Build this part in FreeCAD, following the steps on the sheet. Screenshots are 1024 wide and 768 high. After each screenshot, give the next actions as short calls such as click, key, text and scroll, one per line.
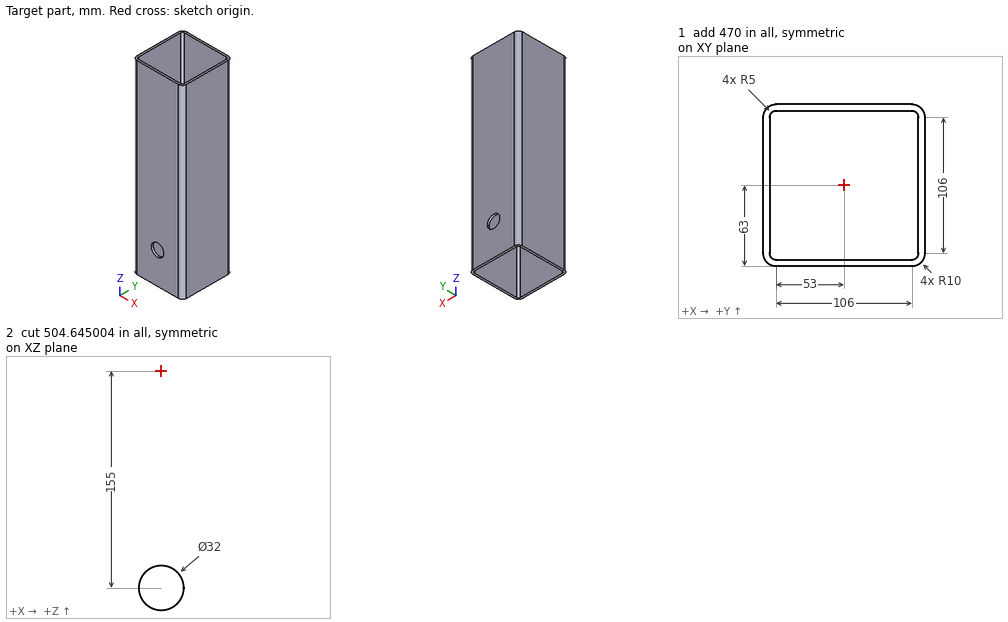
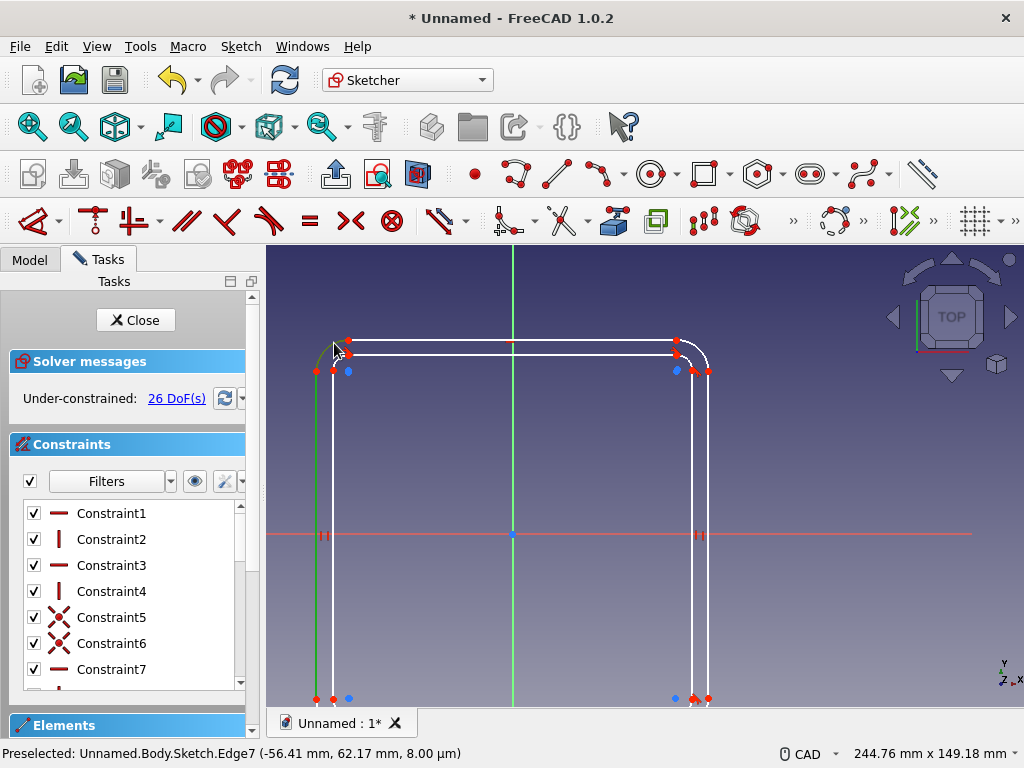
click(269, 222)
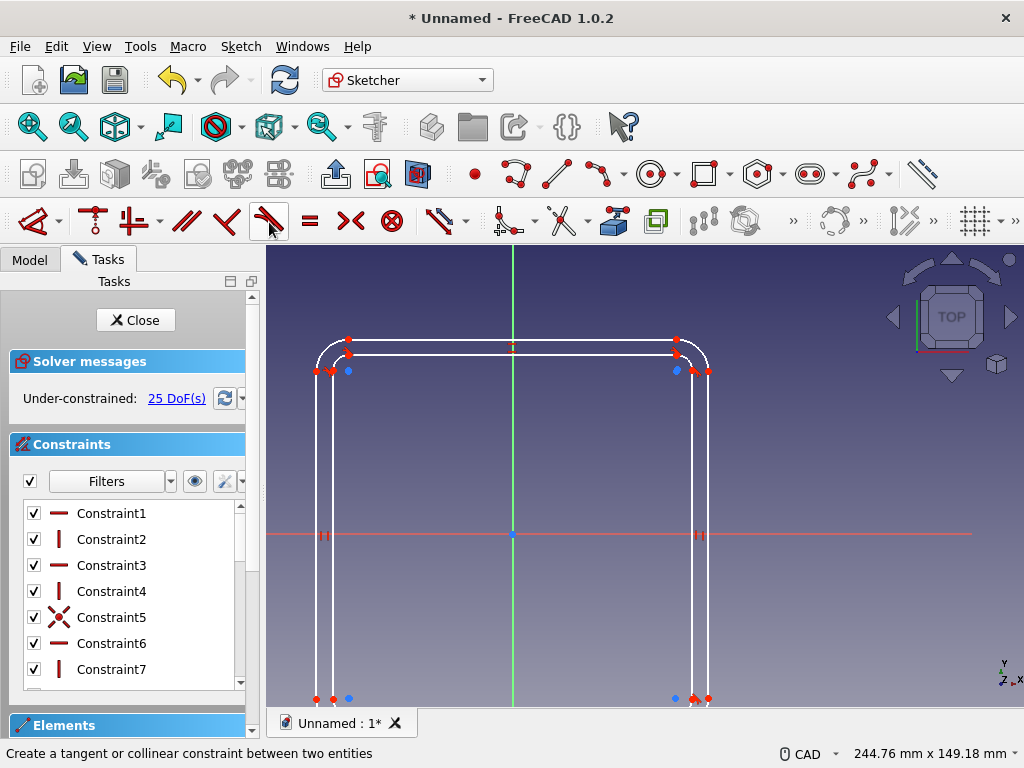
click(316, 470)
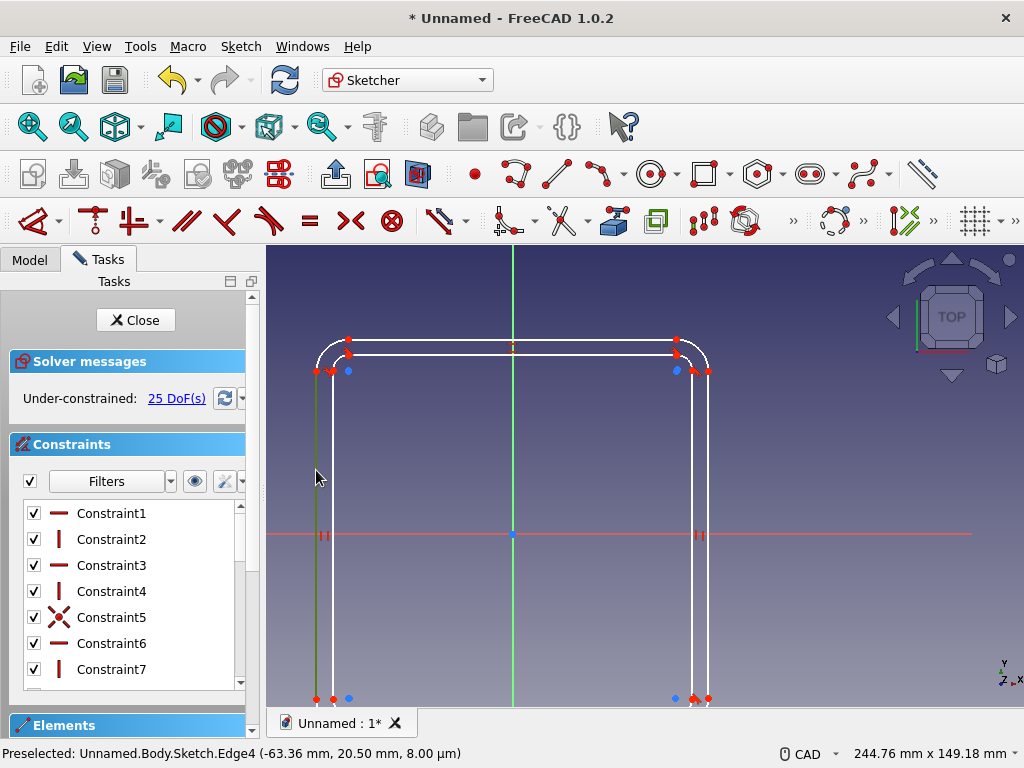
scroll(706, 357, down, 2)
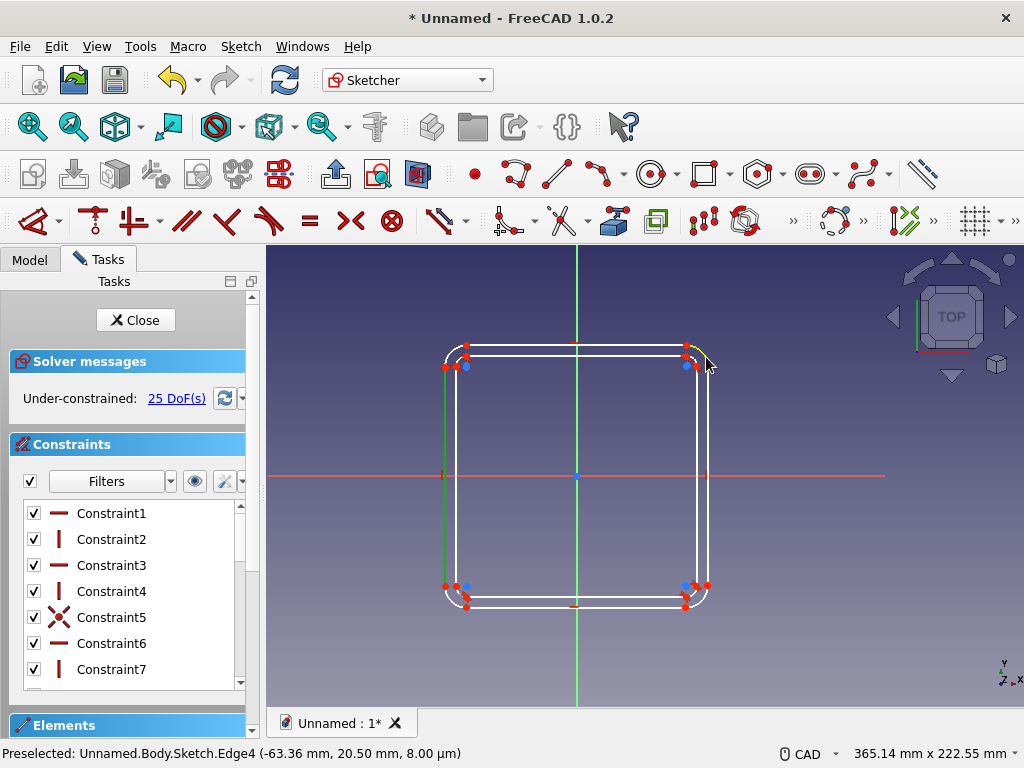
scroll(448, 596, up, 2)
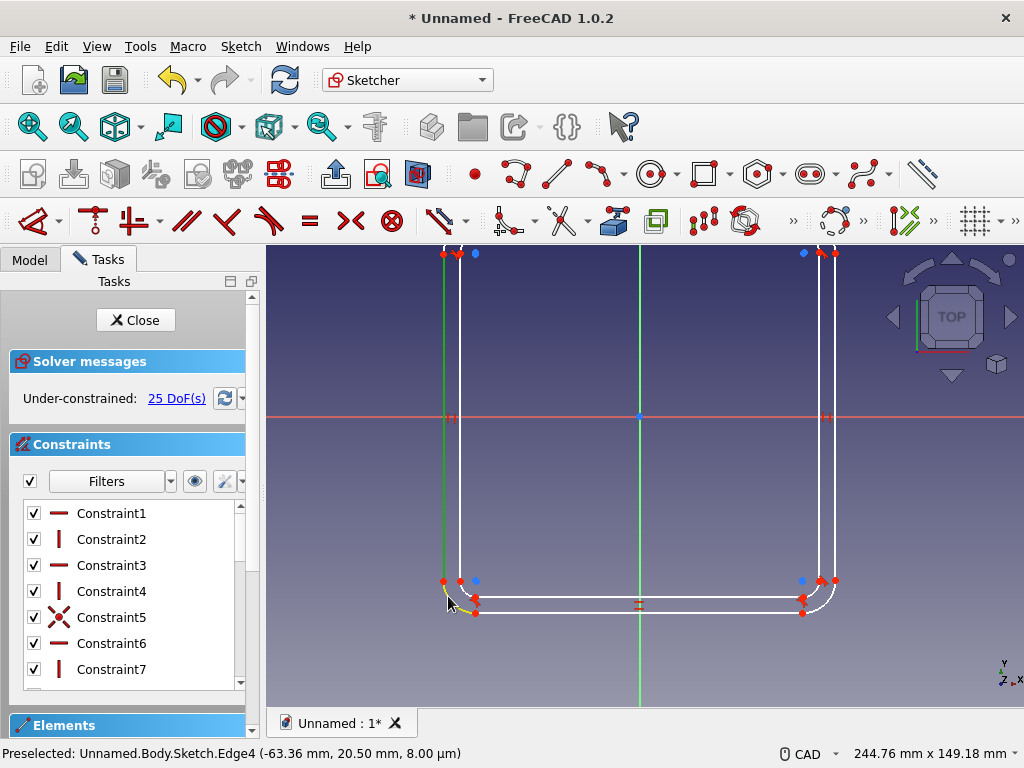
click(447, 596)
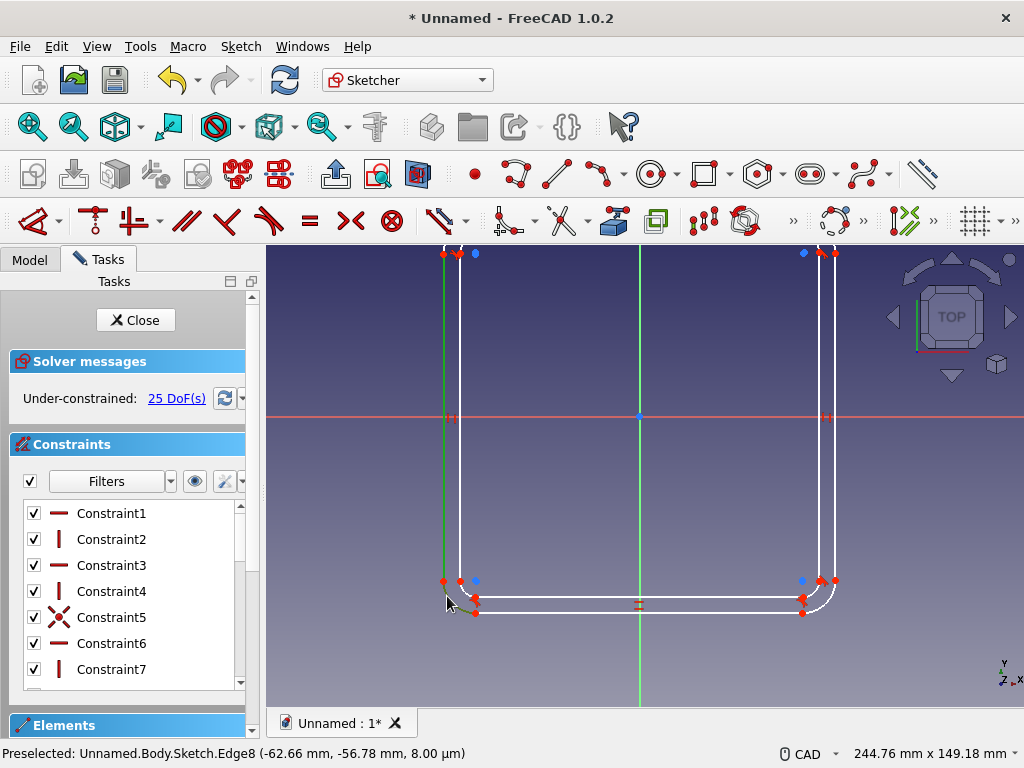
key(t)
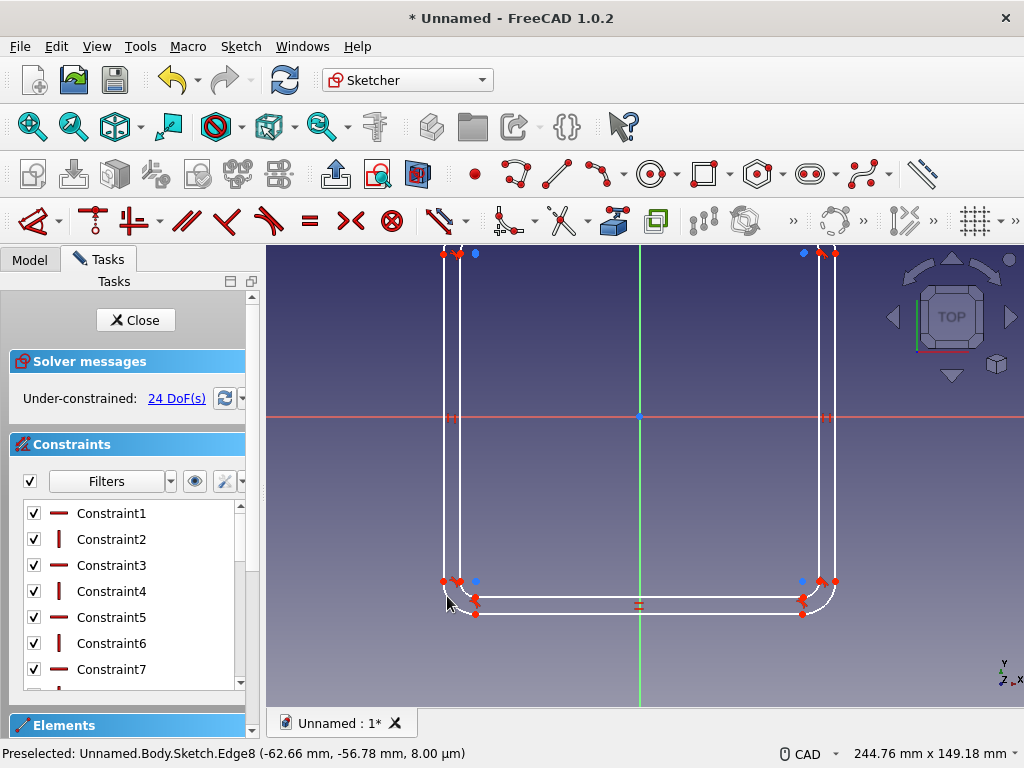
click(705, 597)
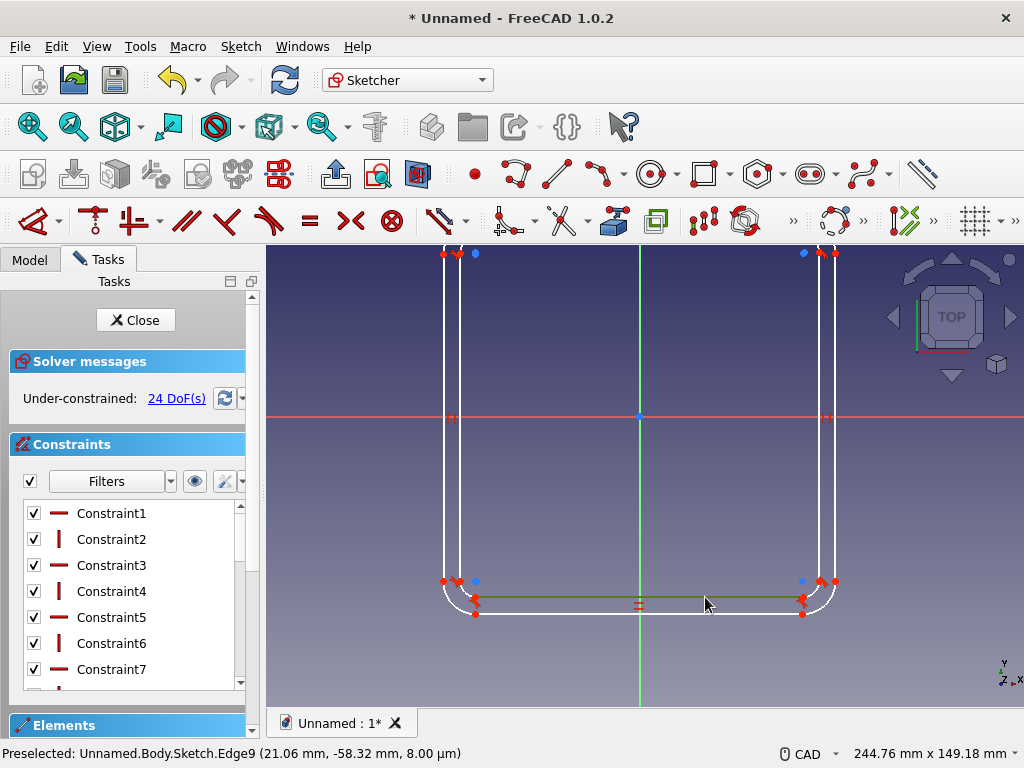
click(465, 593)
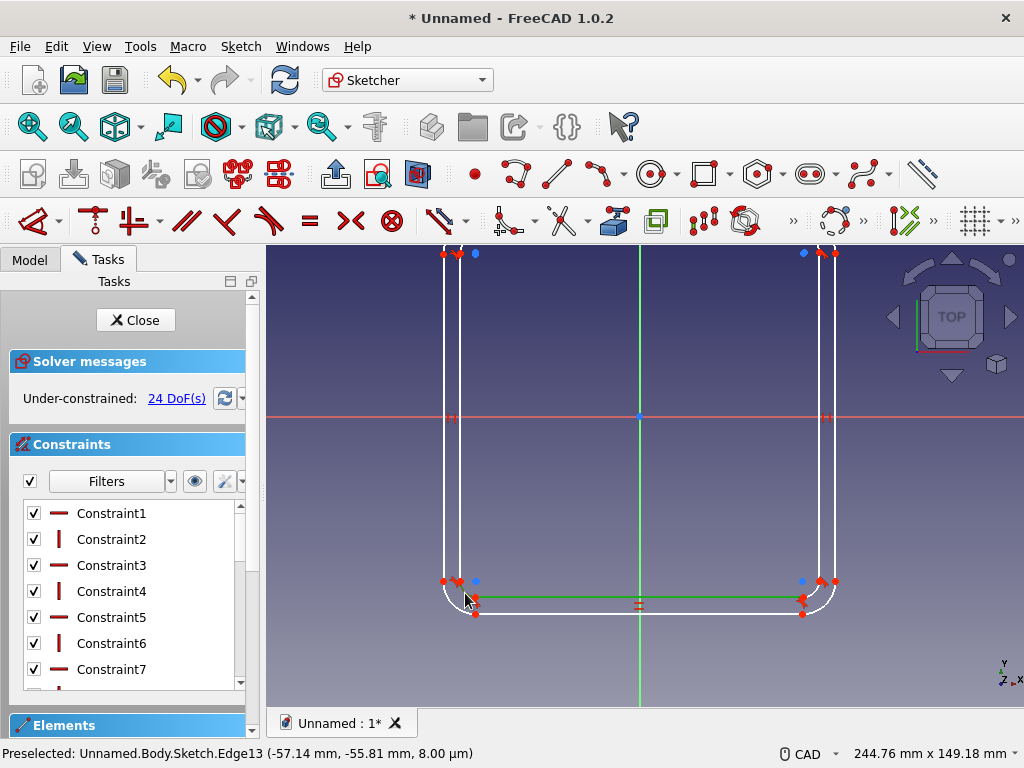
click(269, 222)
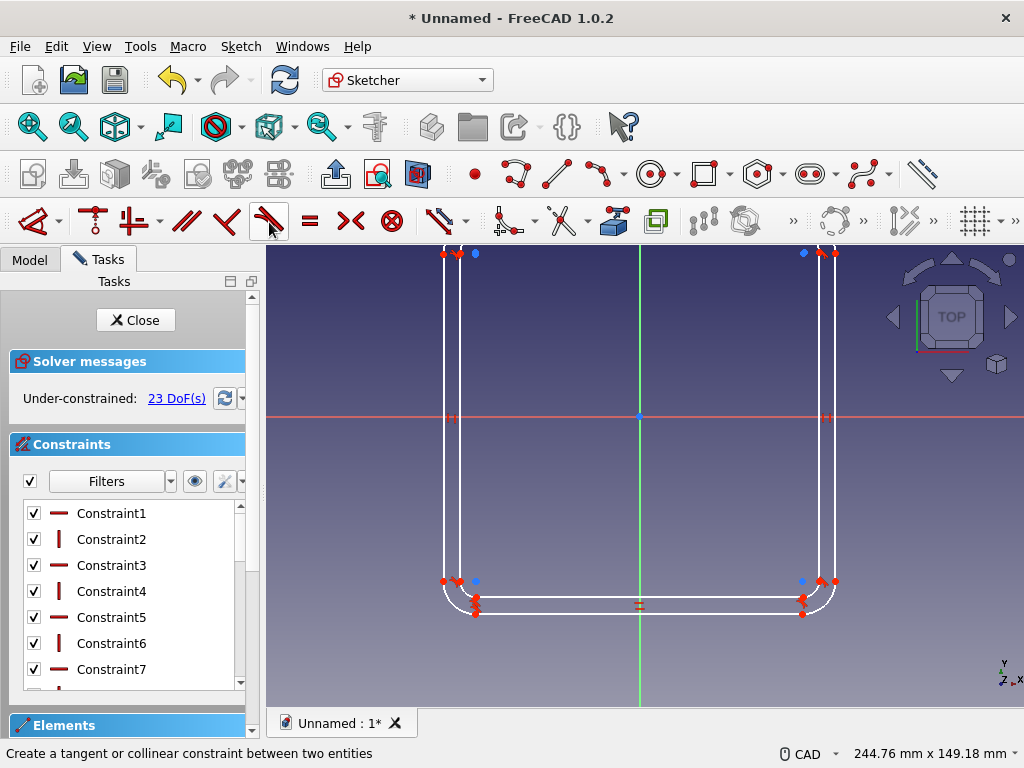
click(705, 597)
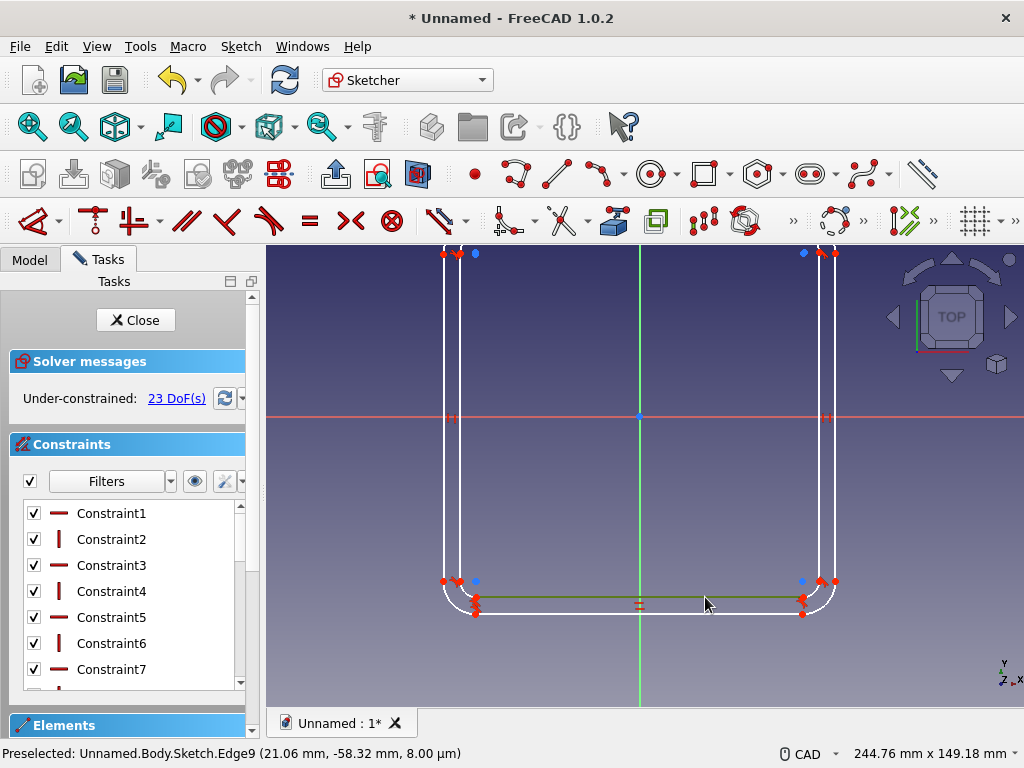
click(814, 593)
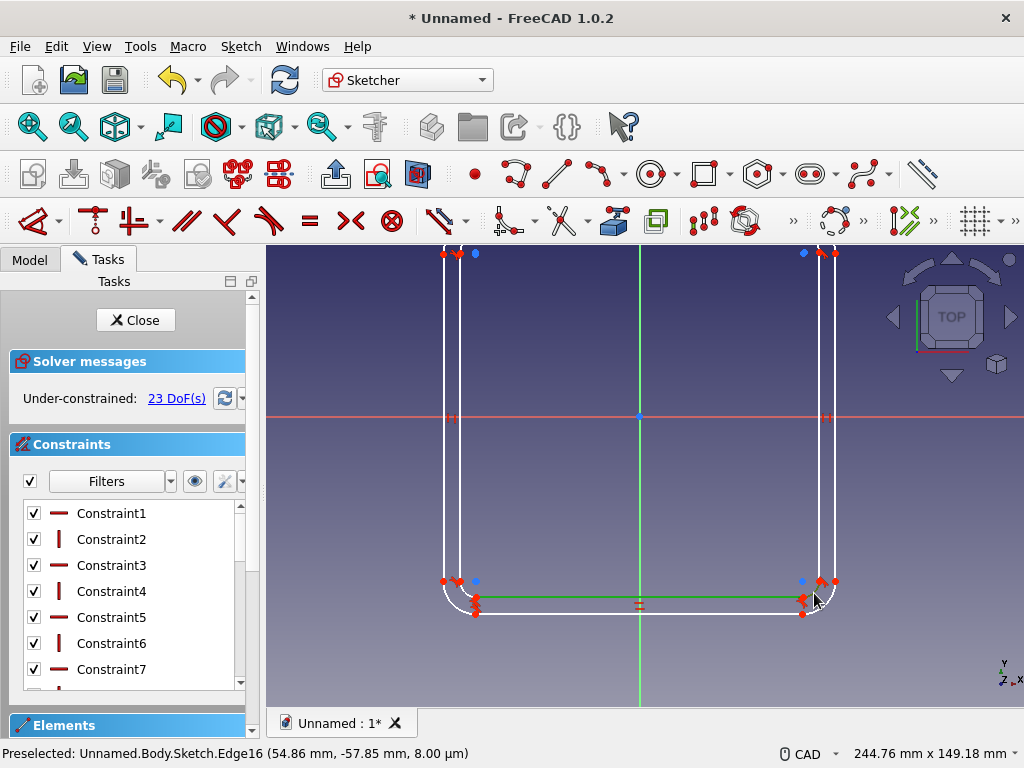
click(269, 222)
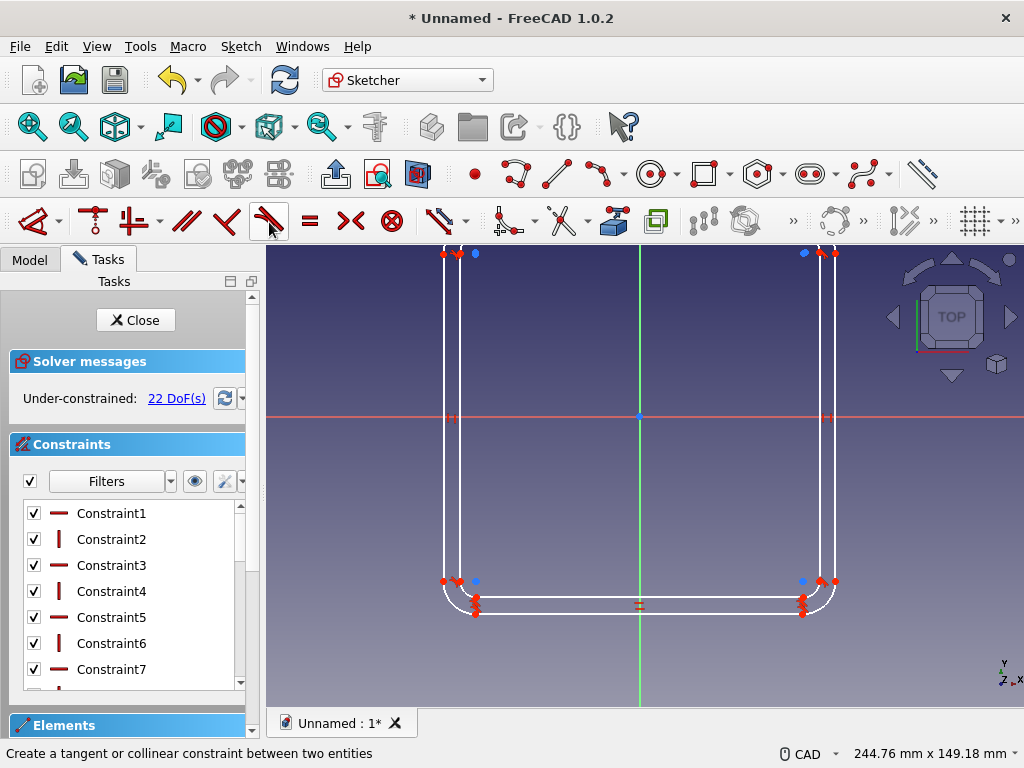
click(460, 483)